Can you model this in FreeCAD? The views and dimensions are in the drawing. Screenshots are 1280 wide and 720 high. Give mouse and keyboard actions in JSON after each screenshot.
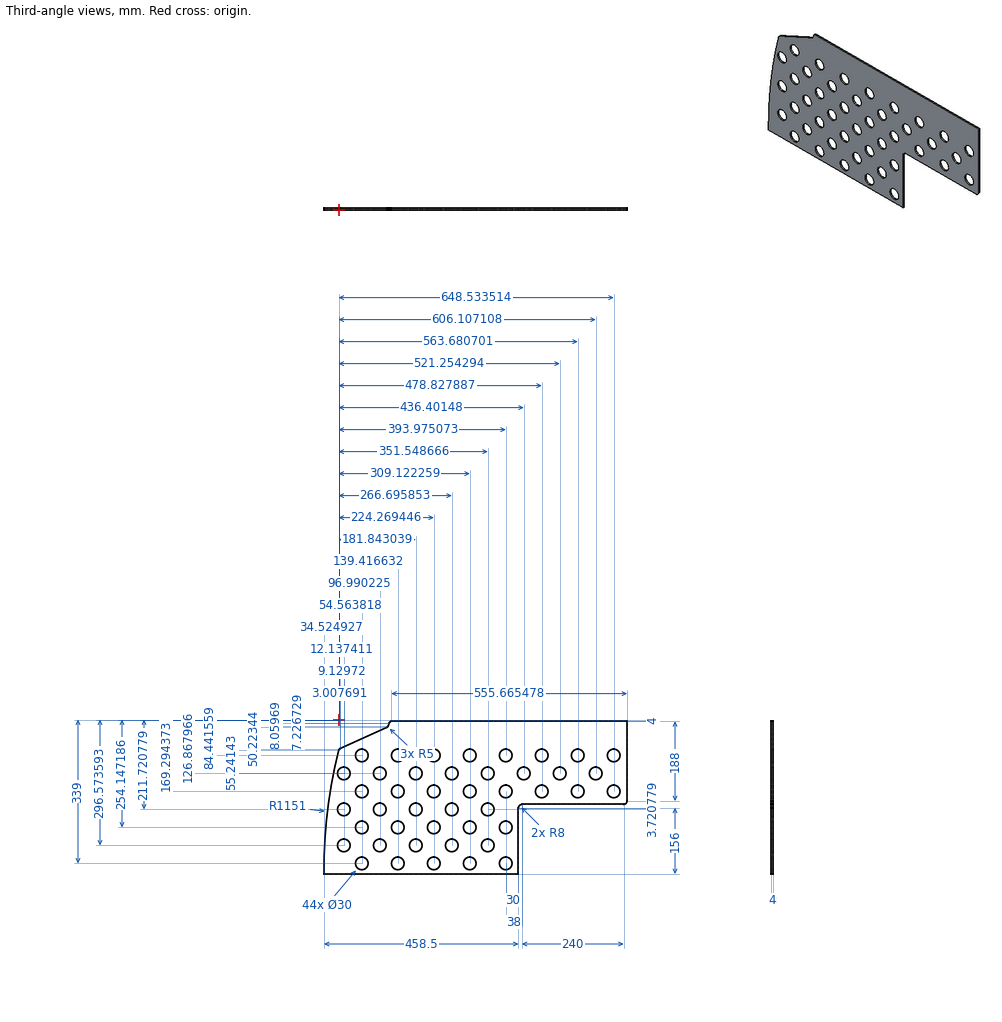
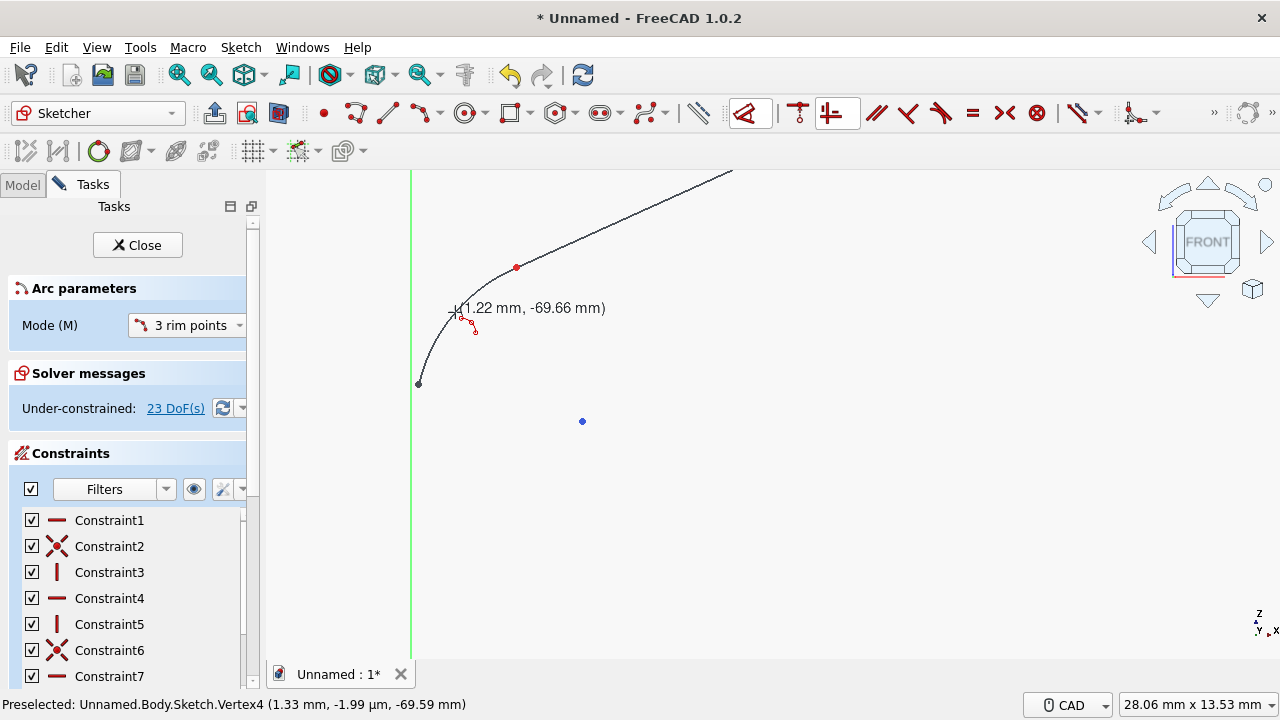
{"action": "scroll", "coordinate": [419, 384], "scroll_direction": "up", "scroll_amount": 4}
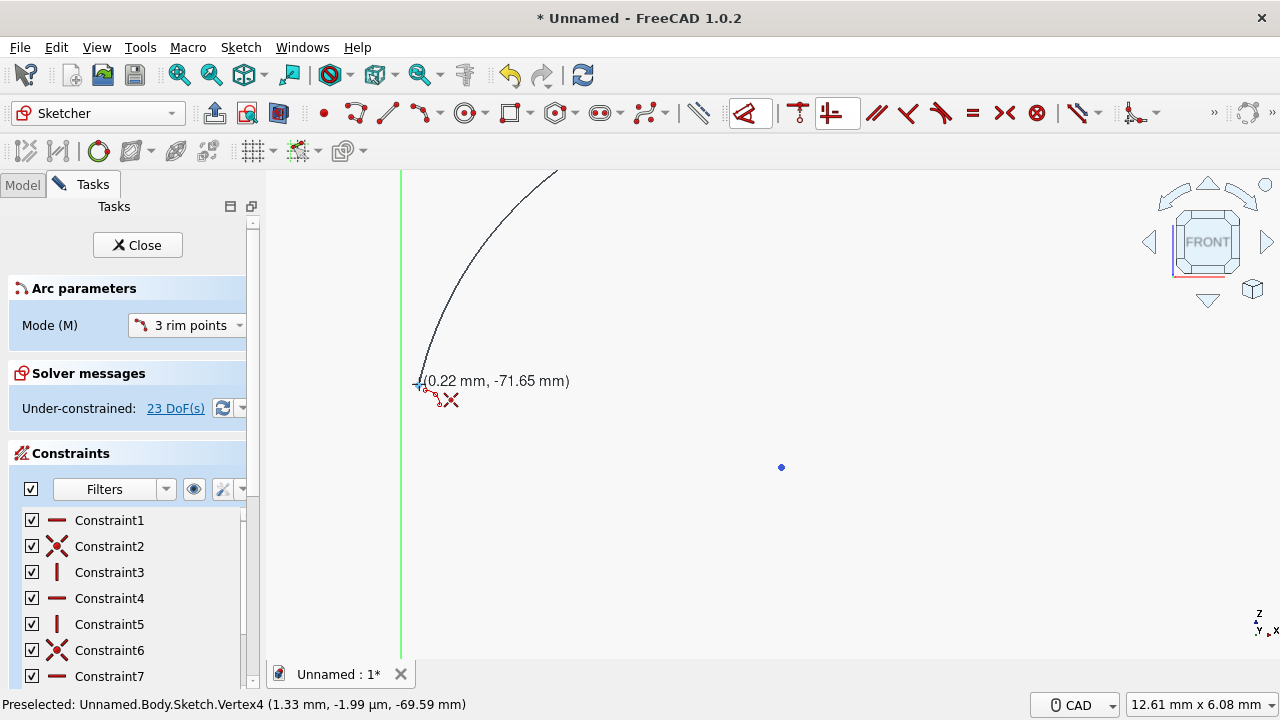
{"action": "left_click", "coordinate": [419, 385]}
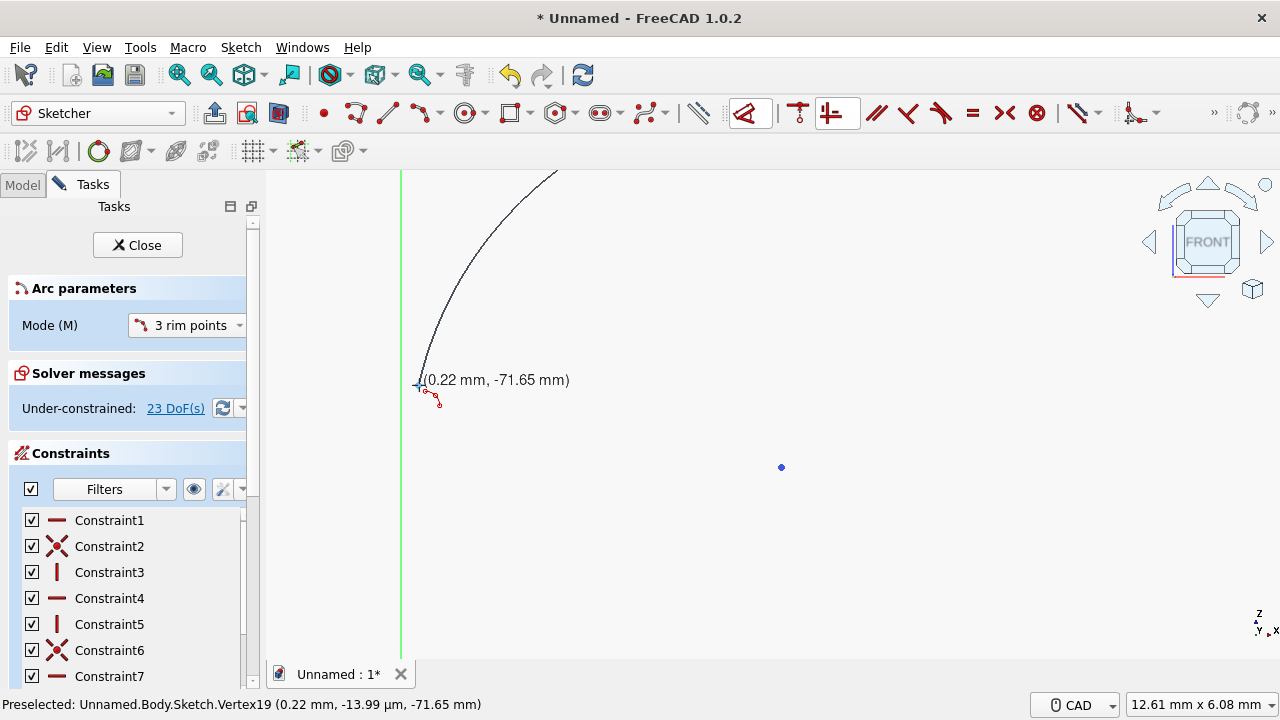
{"action": "scroll", "coordinate": [704, 414], "scroll_direction": "down", "scroll_amount": 15}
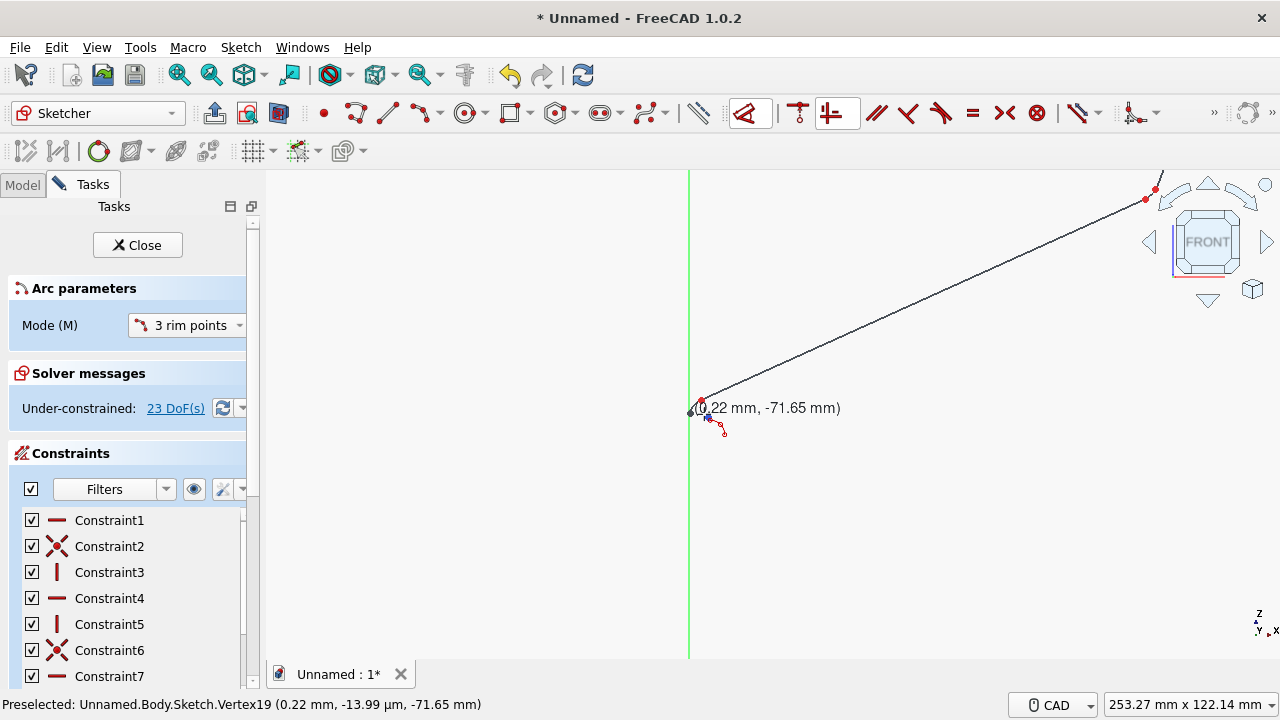
{"action": "scroll", "coordinate": [381, 303], "scroll_direction": "down", "scroll_amount": 8}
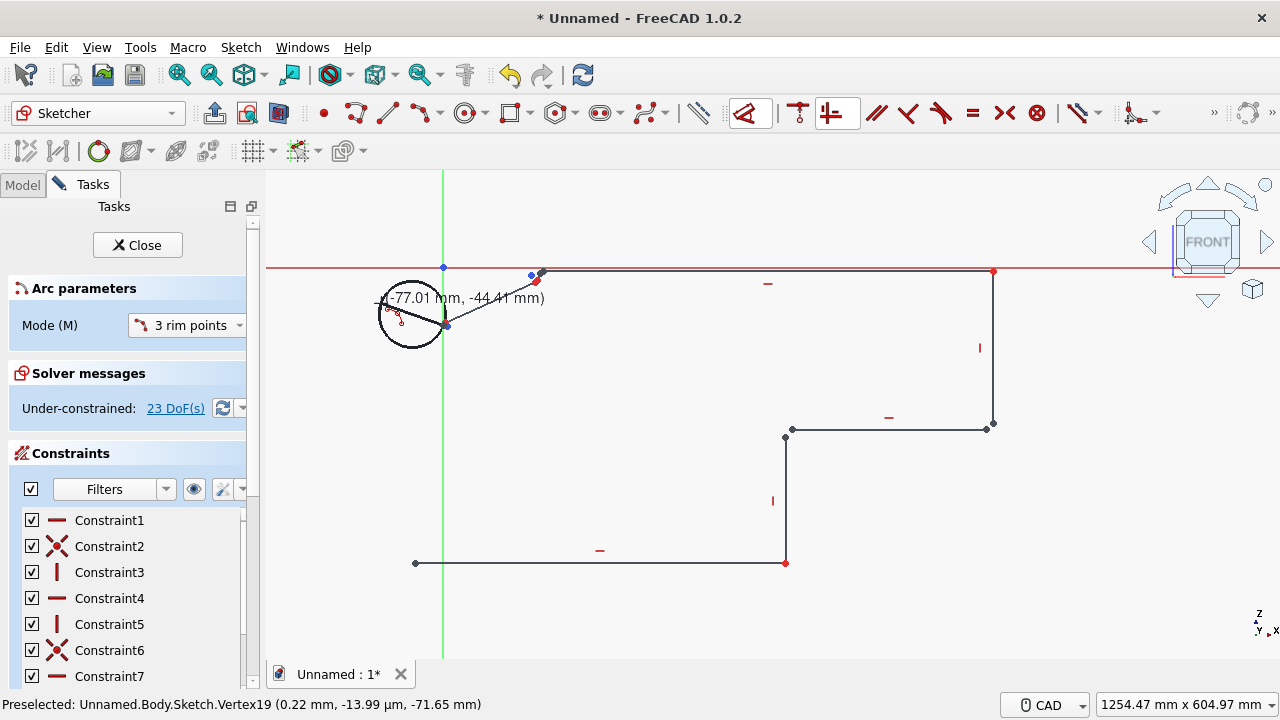
{"action": "left_click", "coordinate": [416, 563]}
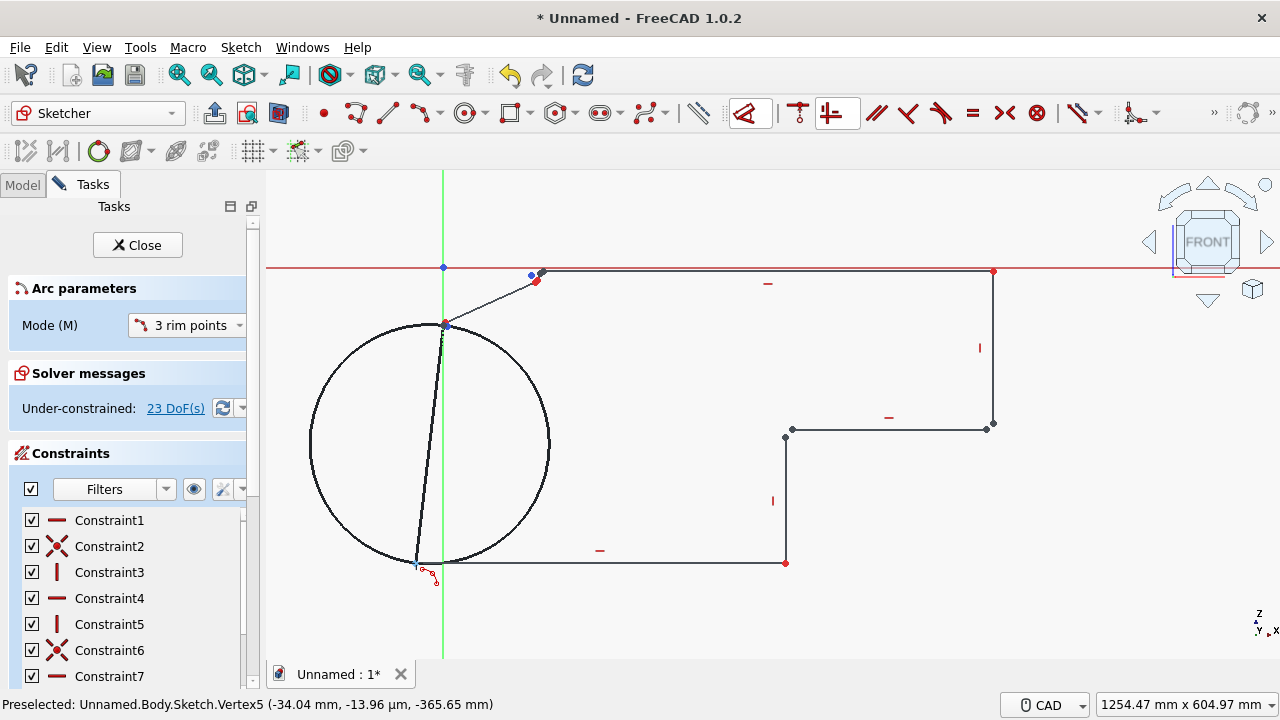
{"action": "scroll", "coordinate": [422, 443], "scroll_direction": "up", "scroll_amount": 4}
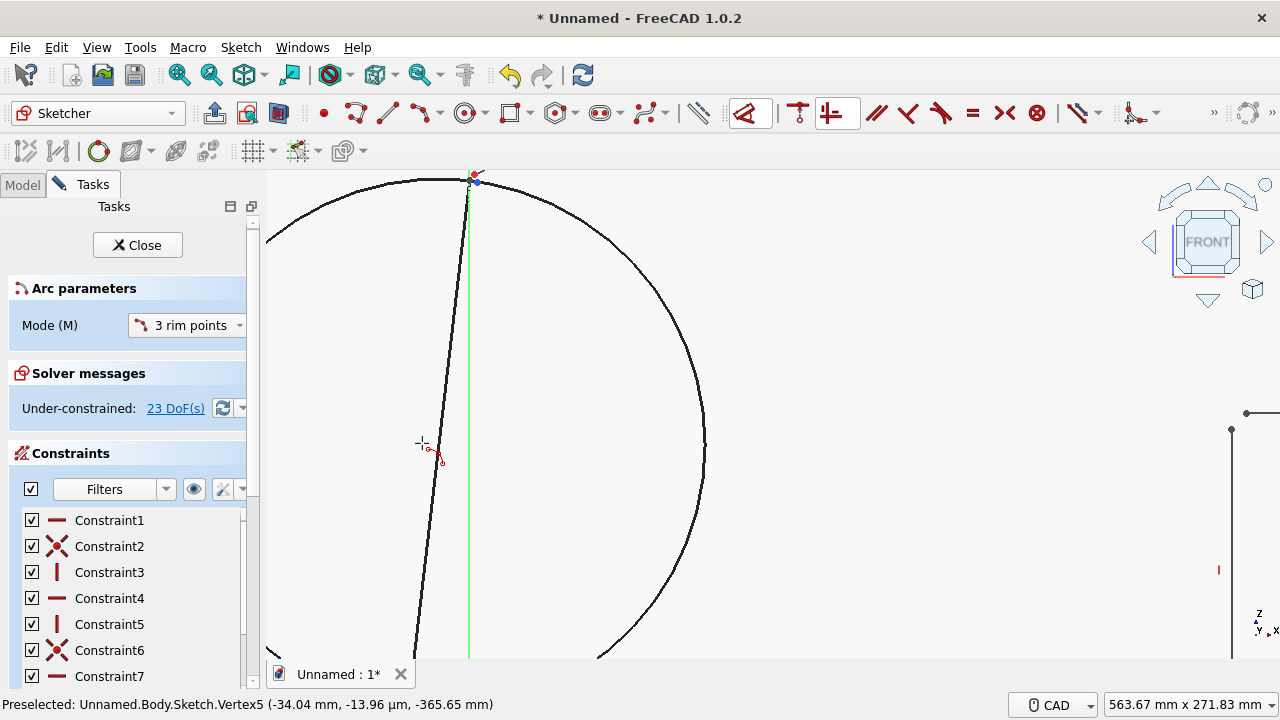
{"action": "left_click", "coordinate": [422, 442]}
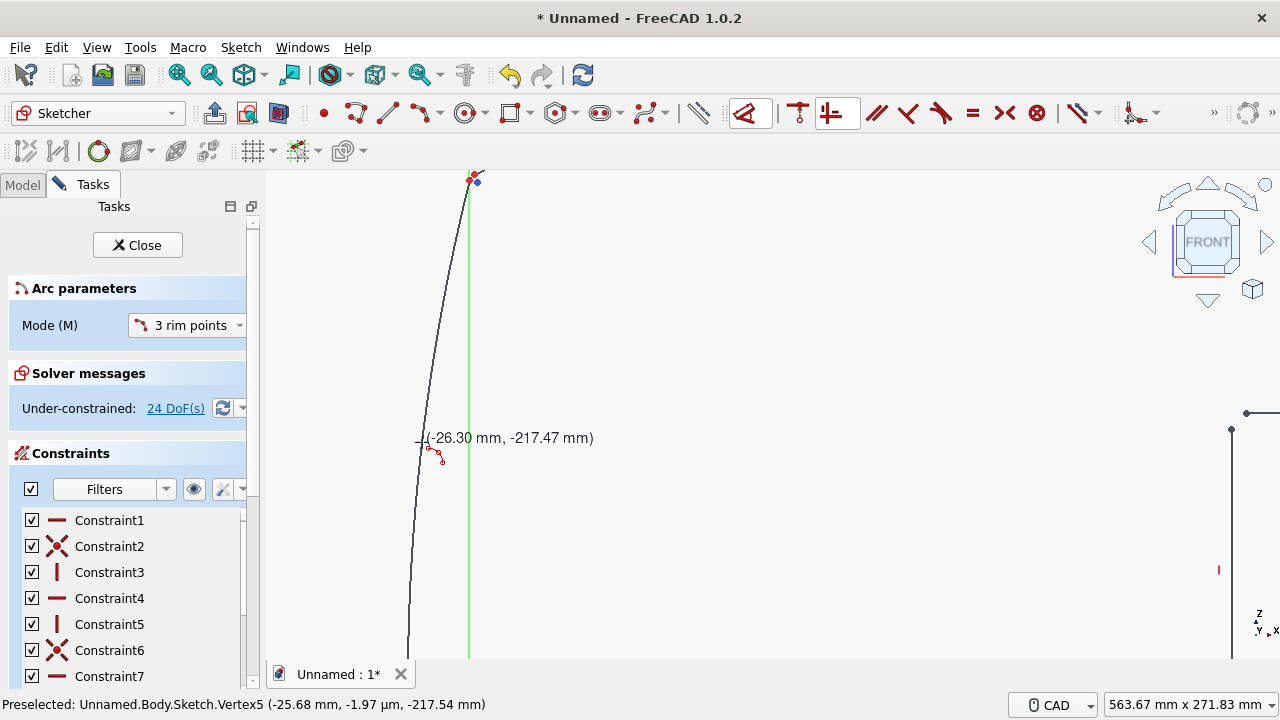
{"action": "scroll", "coordinate": [423, 443], "scroll_direction": "down", "scroll_amount": 4}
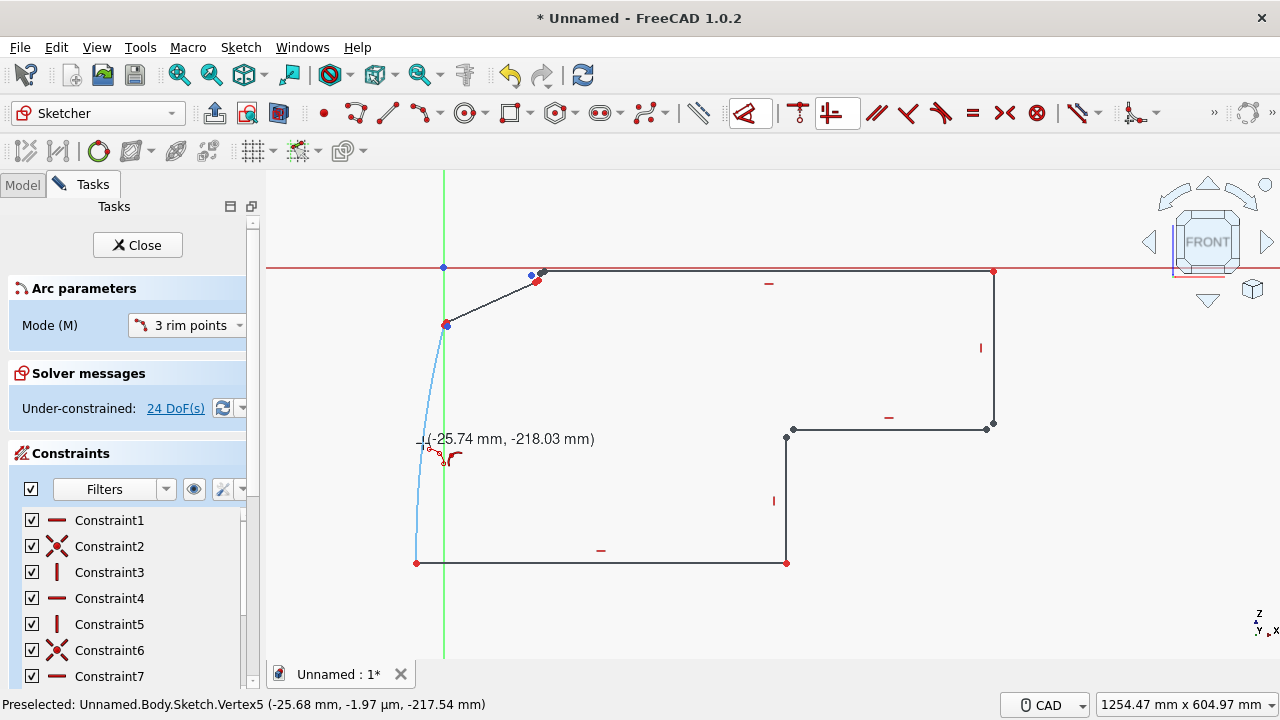
{"action": "scroll", "coordinate": [787, 436], "scroll_direction": "up", "scroll_amount": 3}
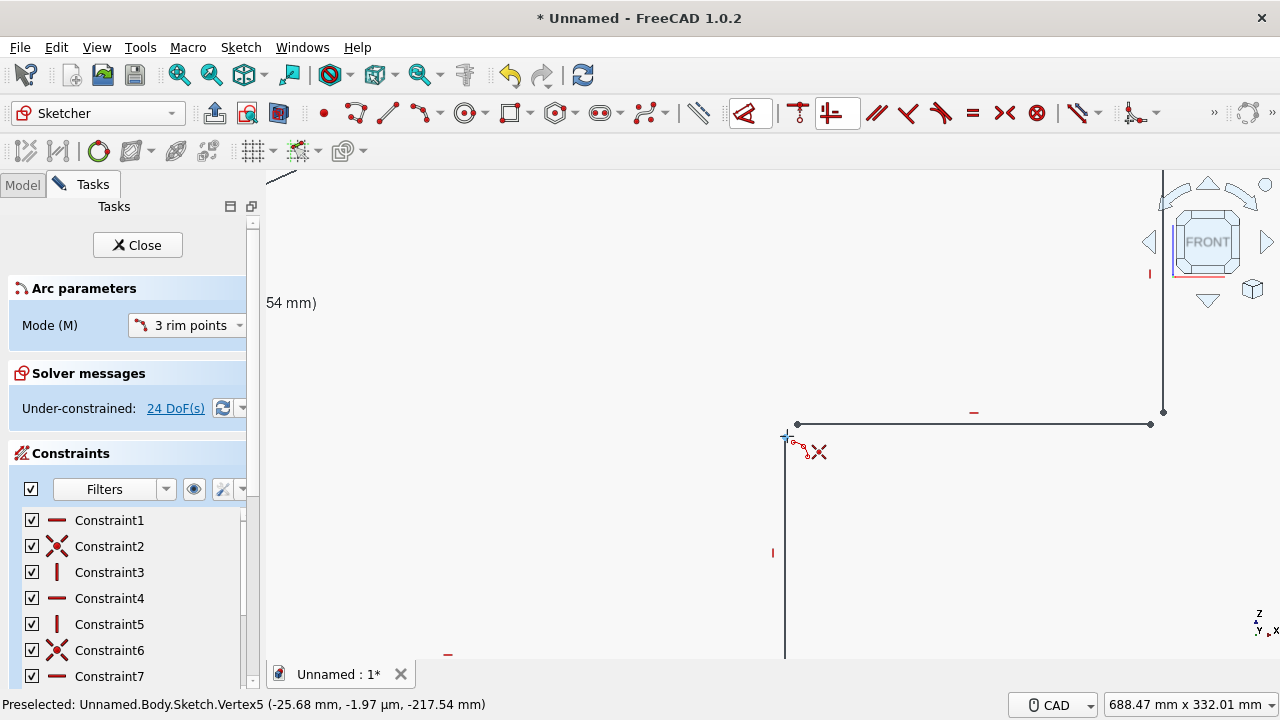
{"action": "left_click", "coordinate": [785, 438]}
{"action": "left_click", "coordinate": [798, 424]}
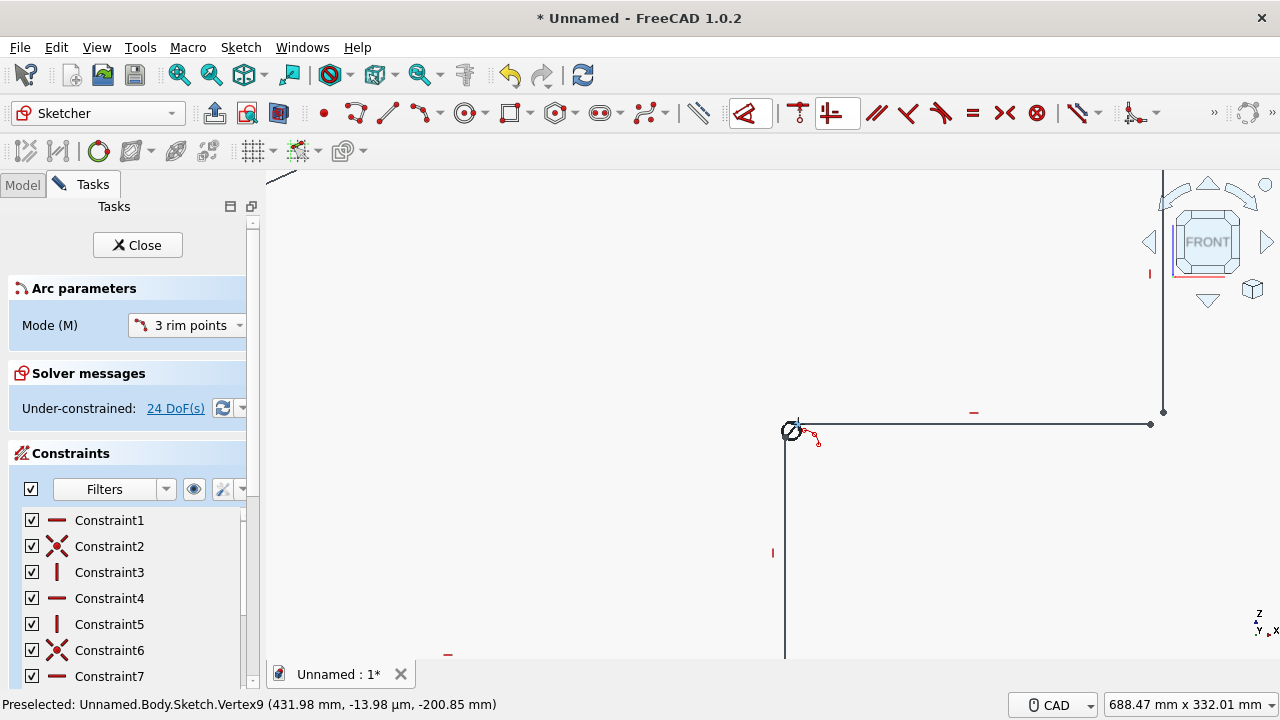
{"action": "scroll", "coordinate": [789, 427], "scroll_direction": "up", "scroll_amount": 8}